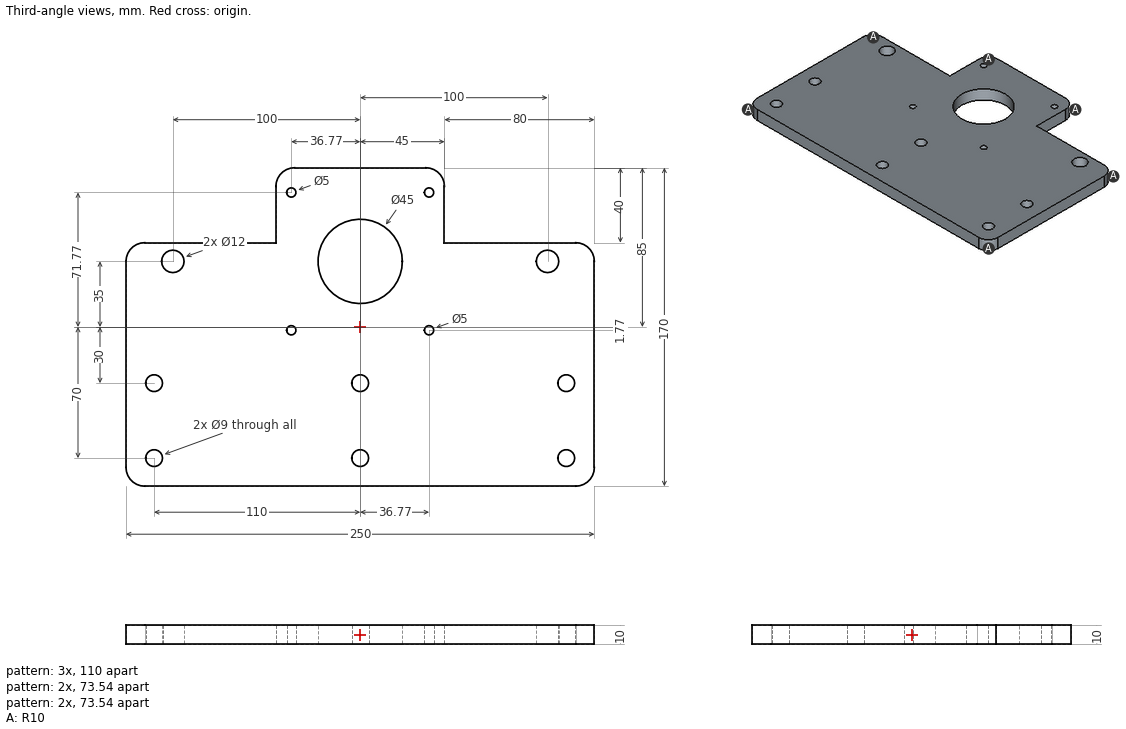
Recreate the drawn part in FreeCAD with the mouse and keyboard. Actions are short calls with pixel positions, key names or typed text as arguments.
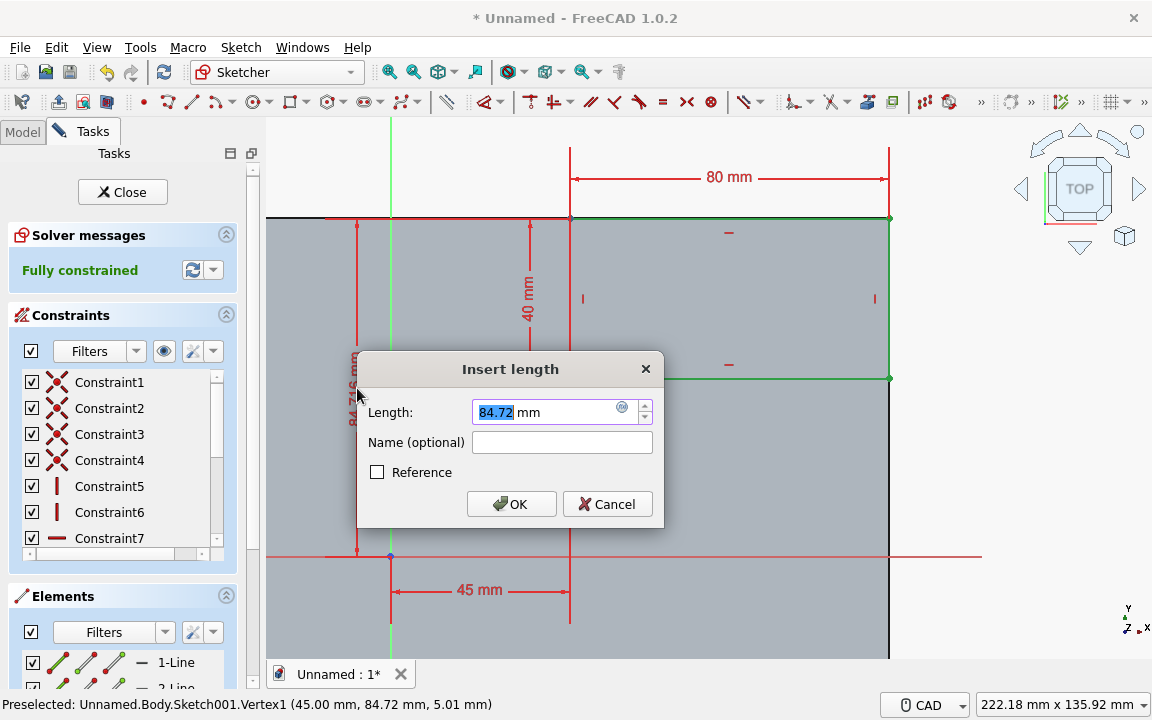
text(85)
key(Return)
key(Escape)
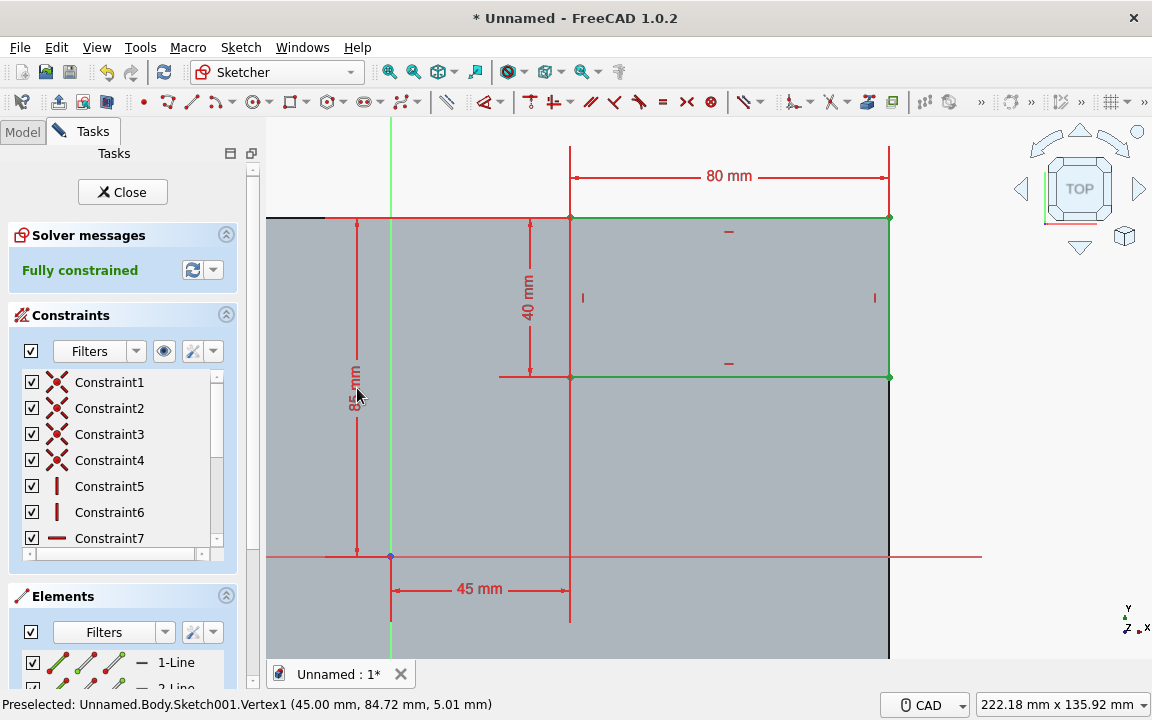
click(123, 192)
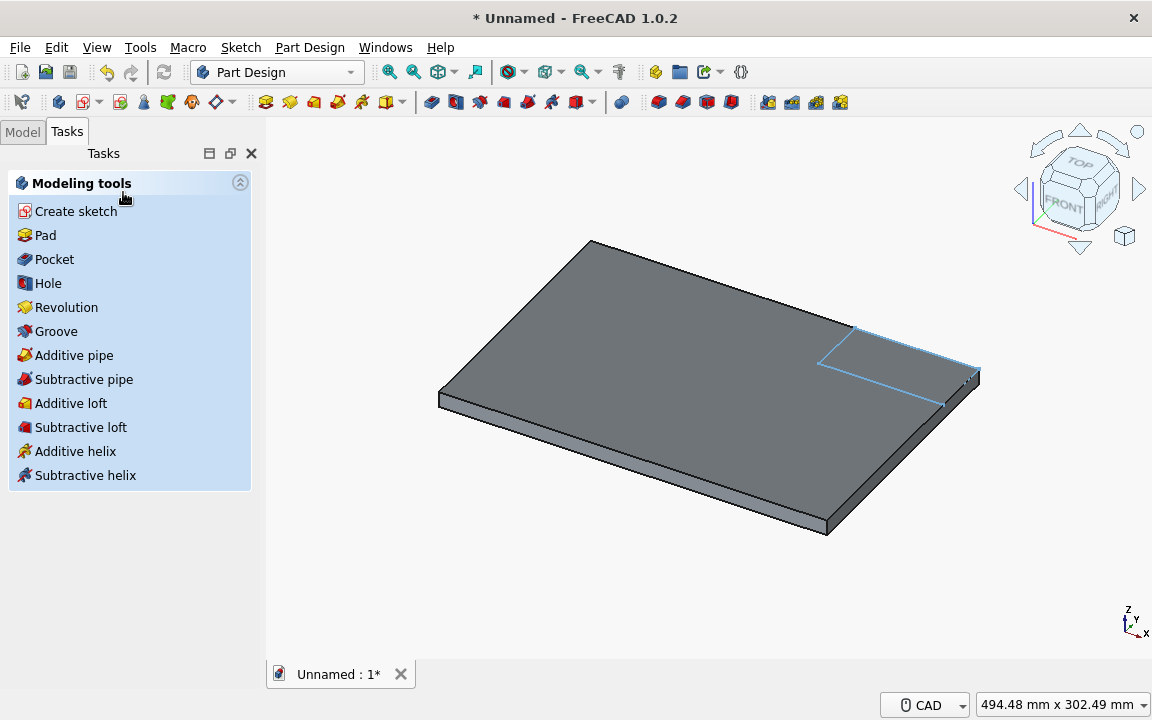
click(432, 102)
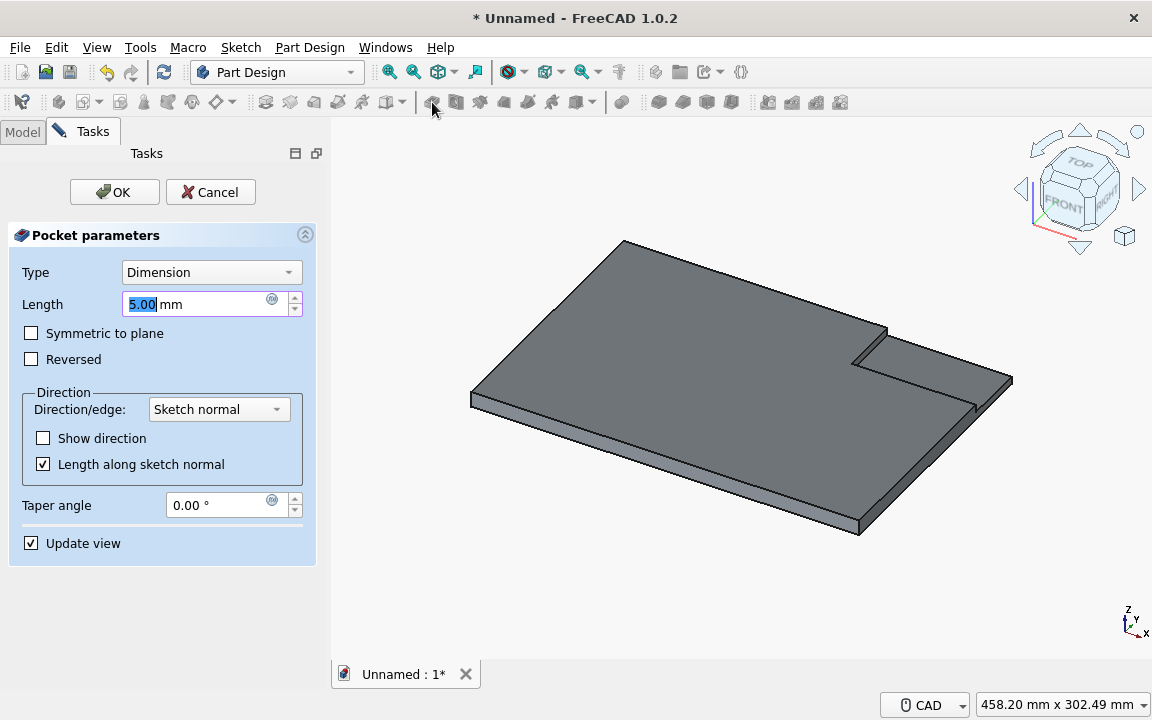
text(10)
key(Tab)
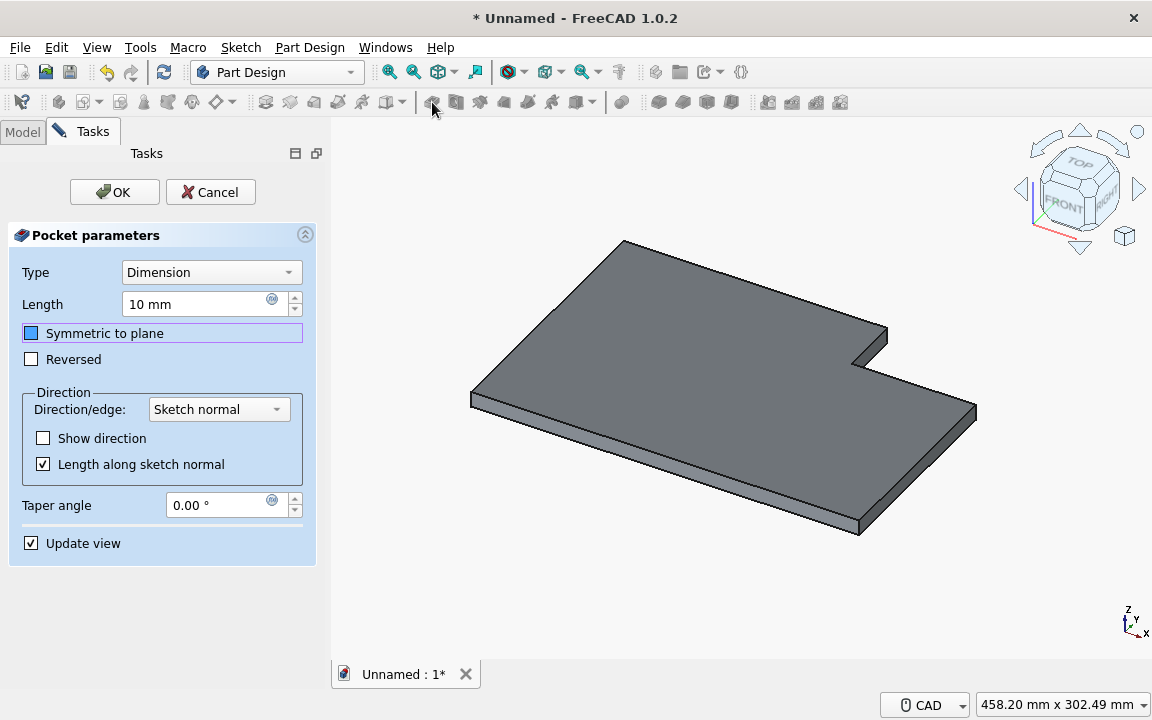
click(115, 192)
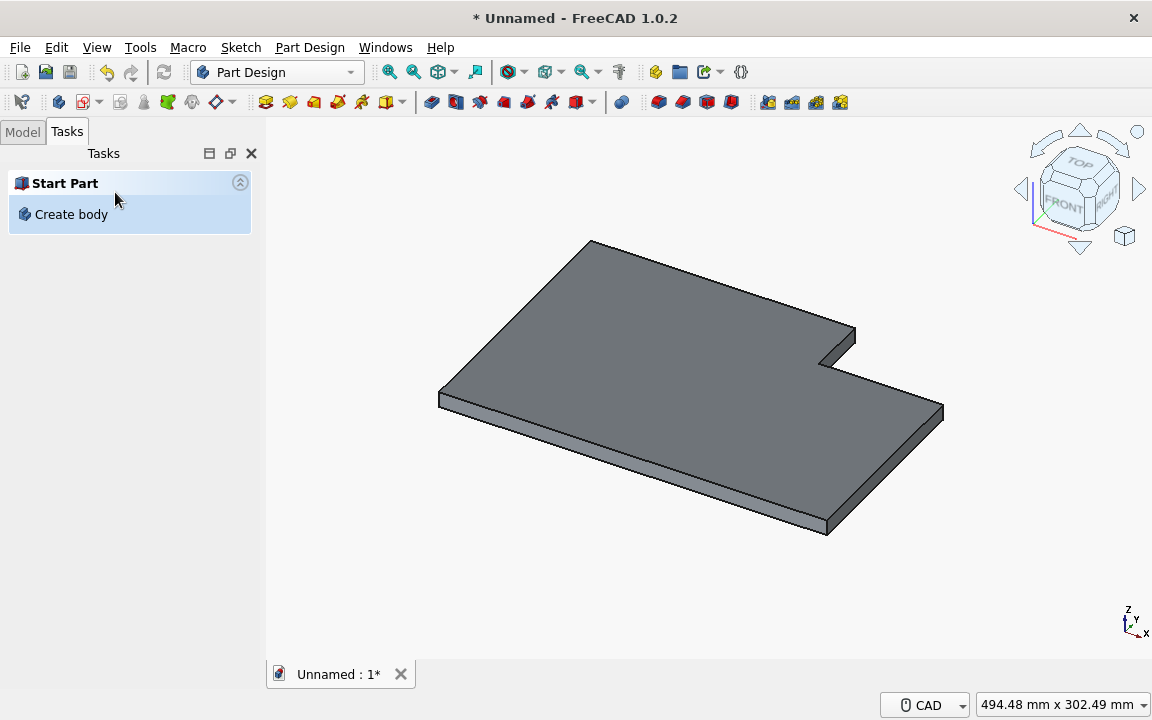
click(23, 131)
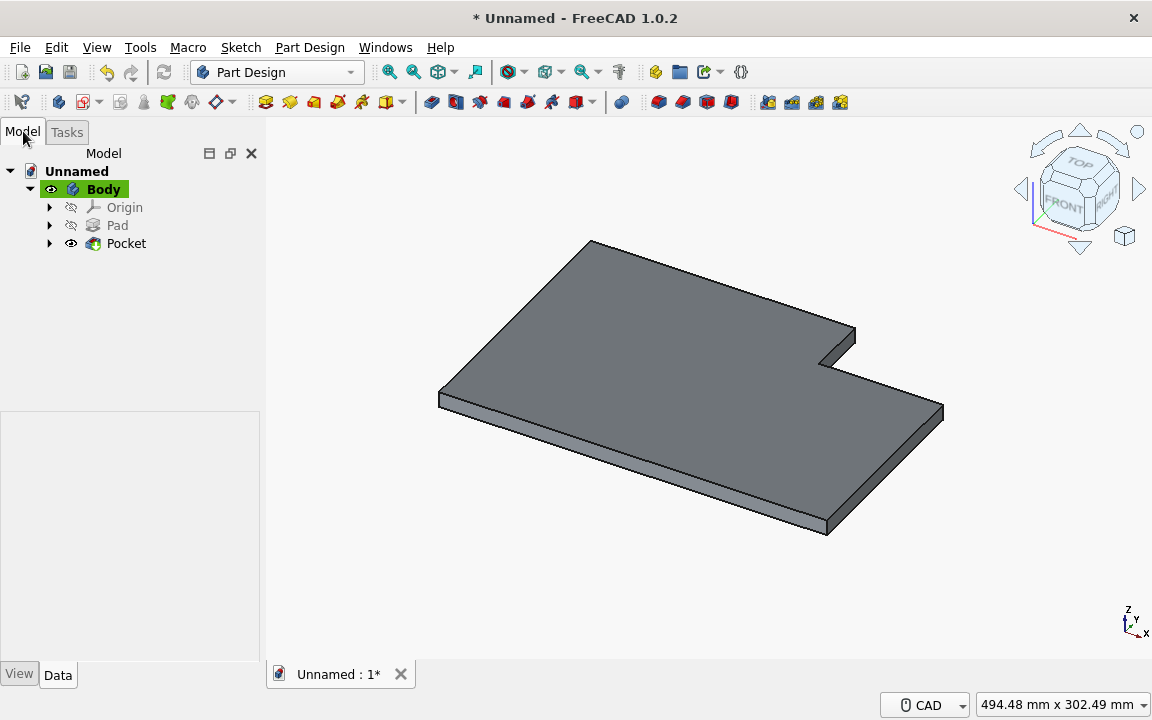
click(116, 243)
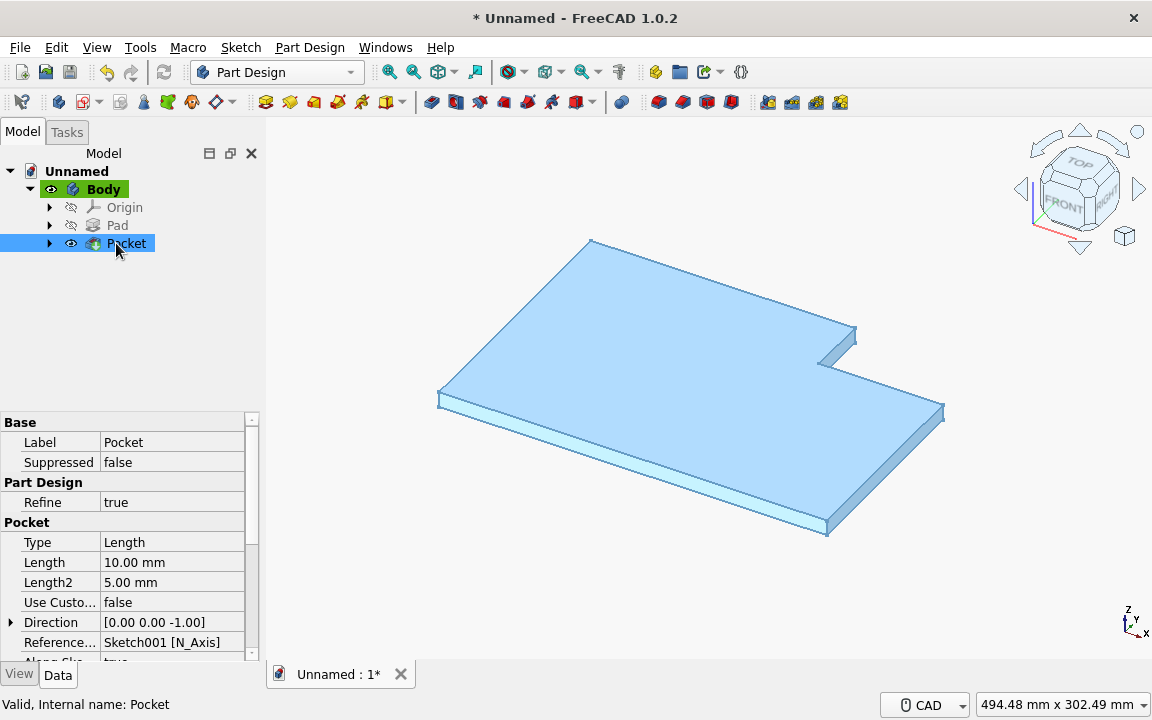
click(768, 102)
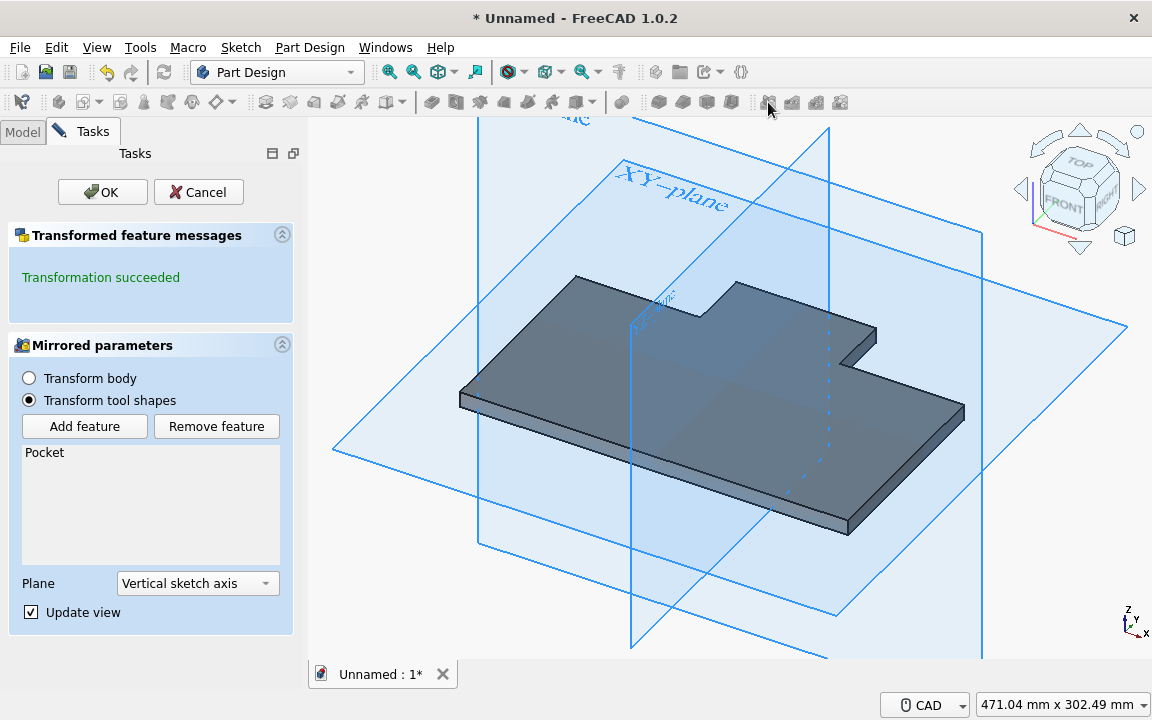
click(198, 584)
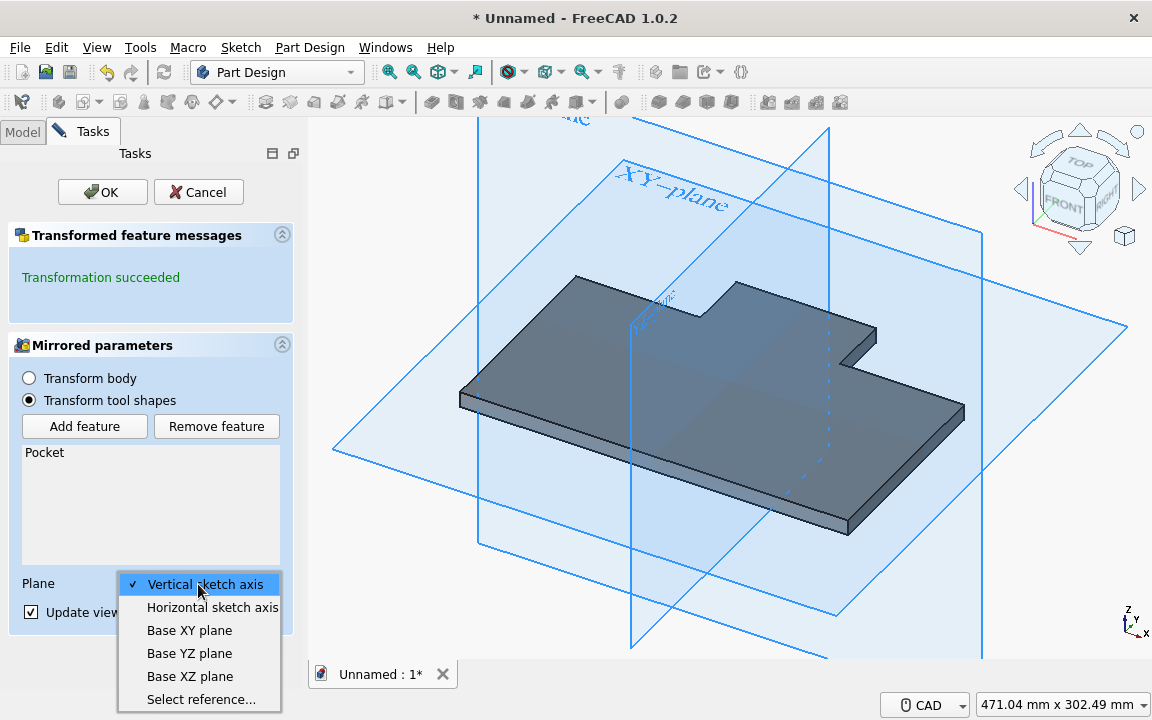
click(198, 654)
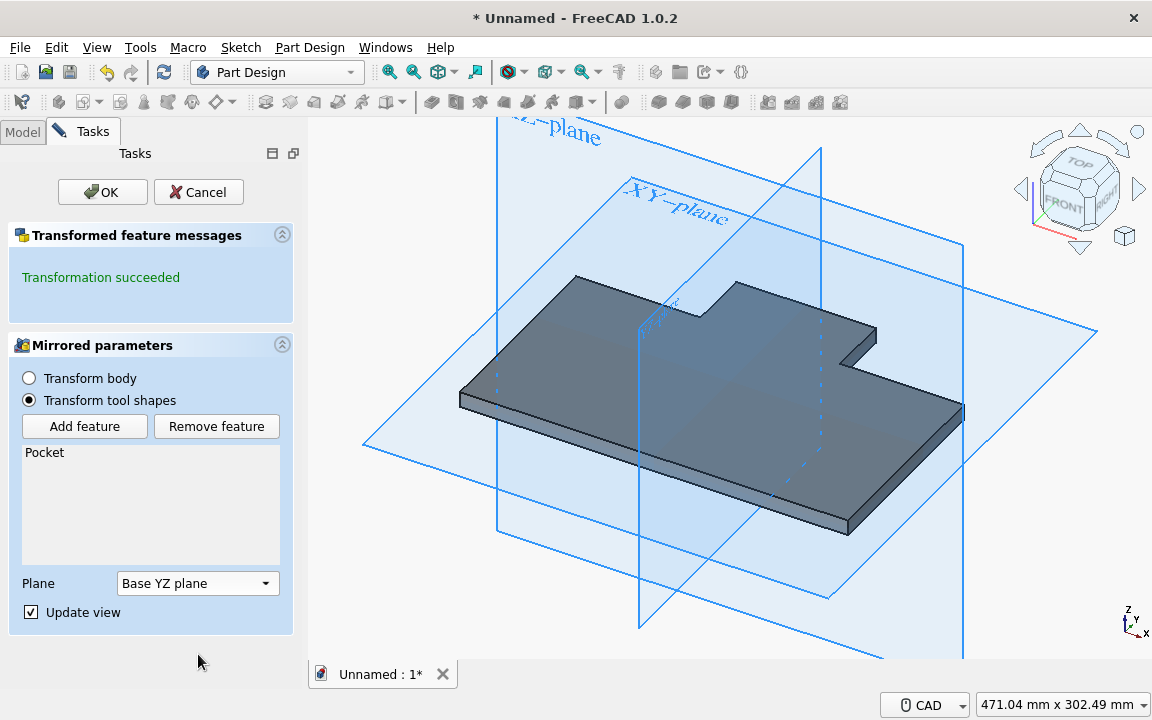
click(103, 192)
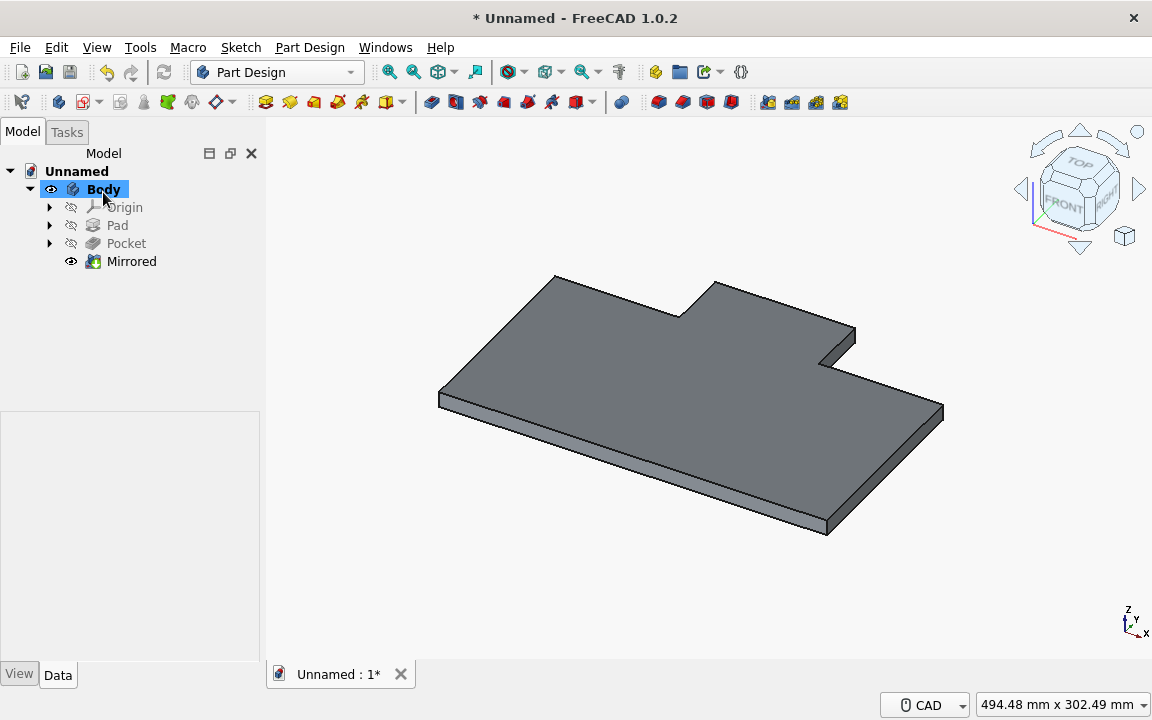
click(709, 380)